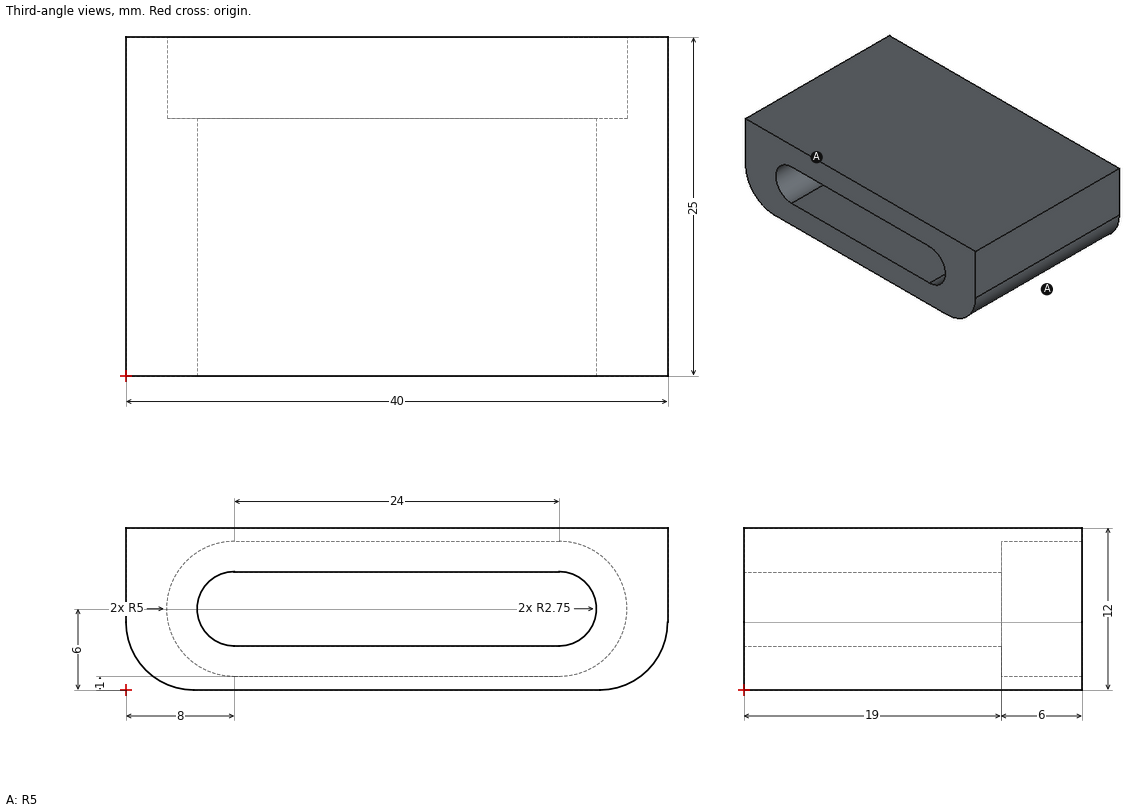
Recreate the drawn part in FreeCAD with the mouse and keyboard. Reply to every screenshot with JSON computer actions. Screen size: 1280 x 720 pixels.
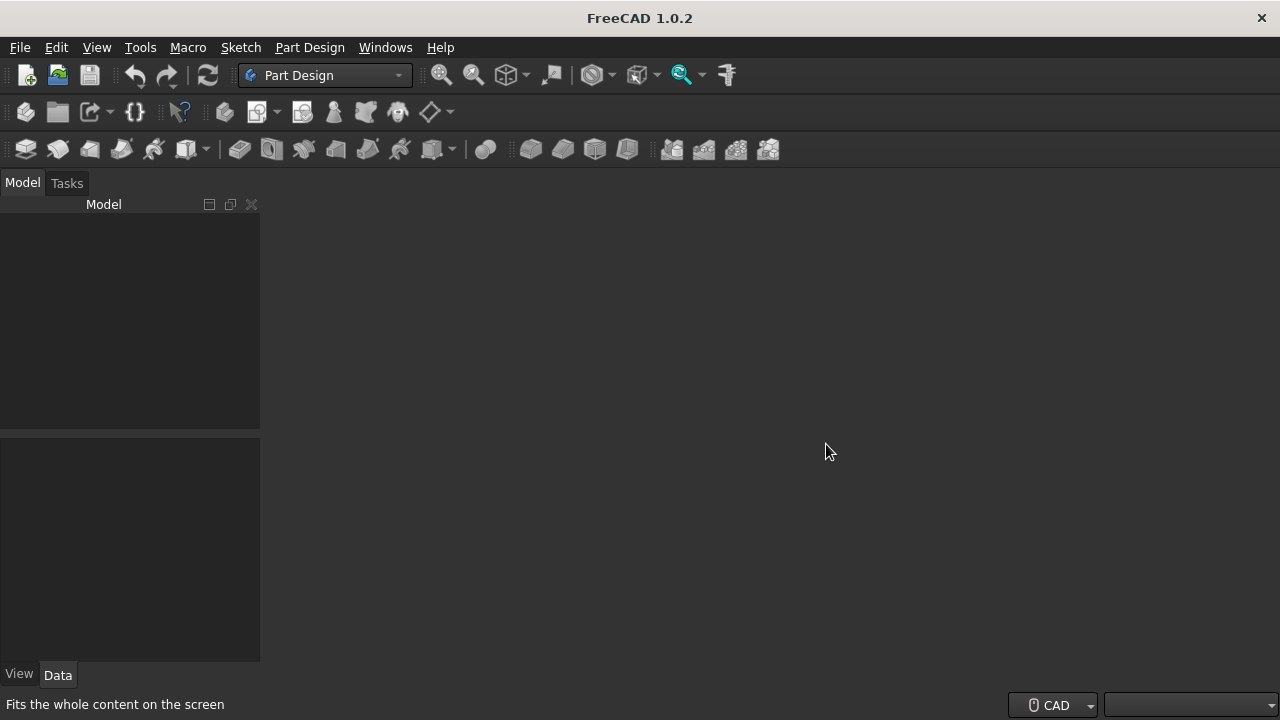
{"action": "key", "text": "ctrl+n"}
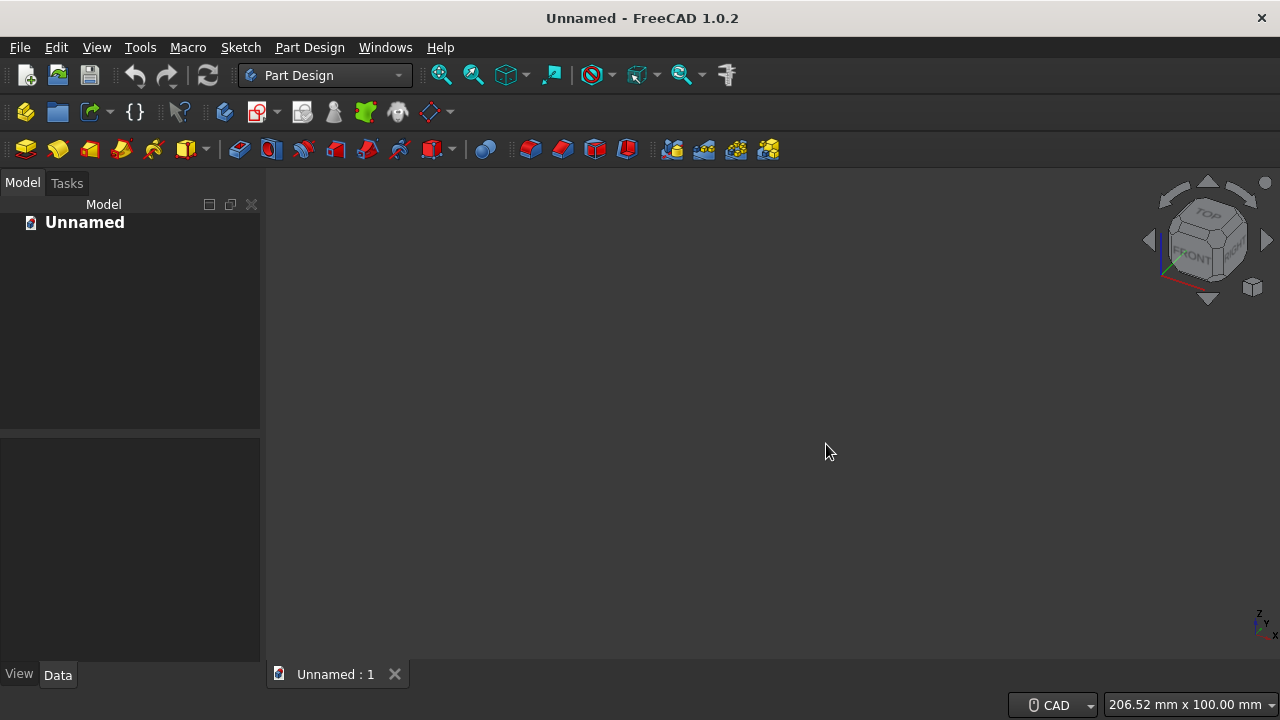
{"action": "left_click", "coordinate": [258, 112]}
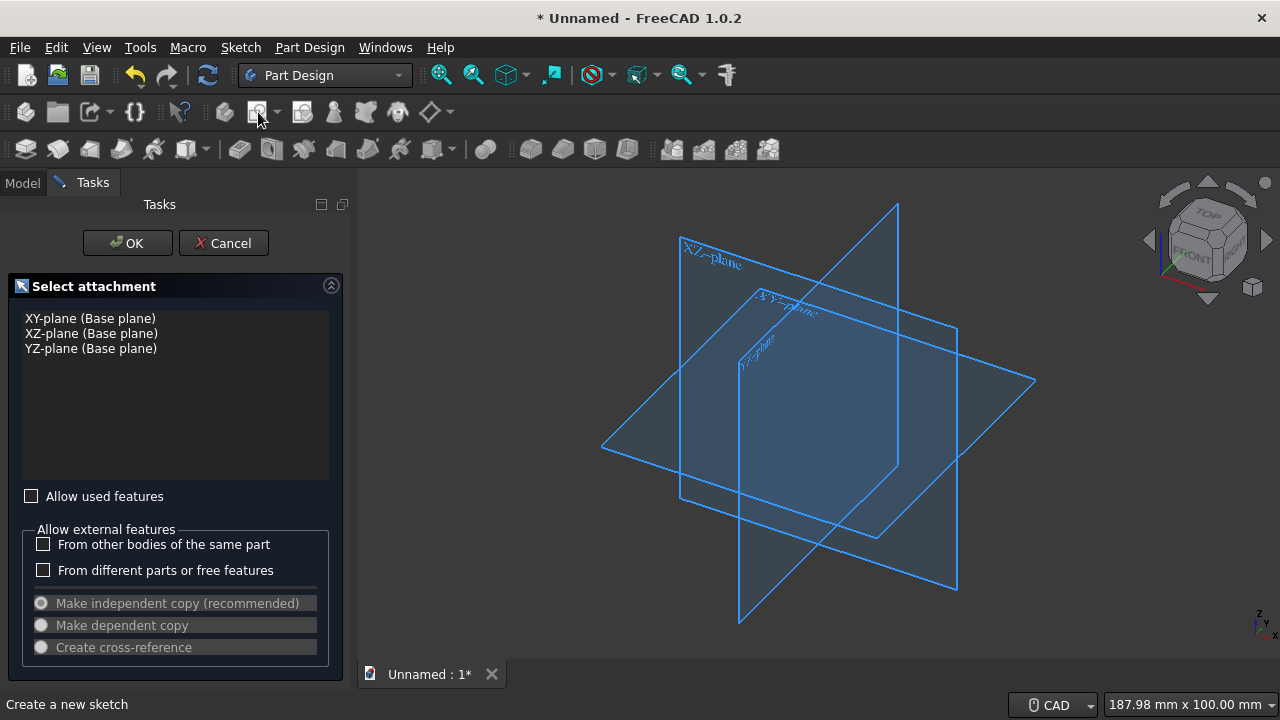
{"action": "left_click", "coordinate": [82, 318]}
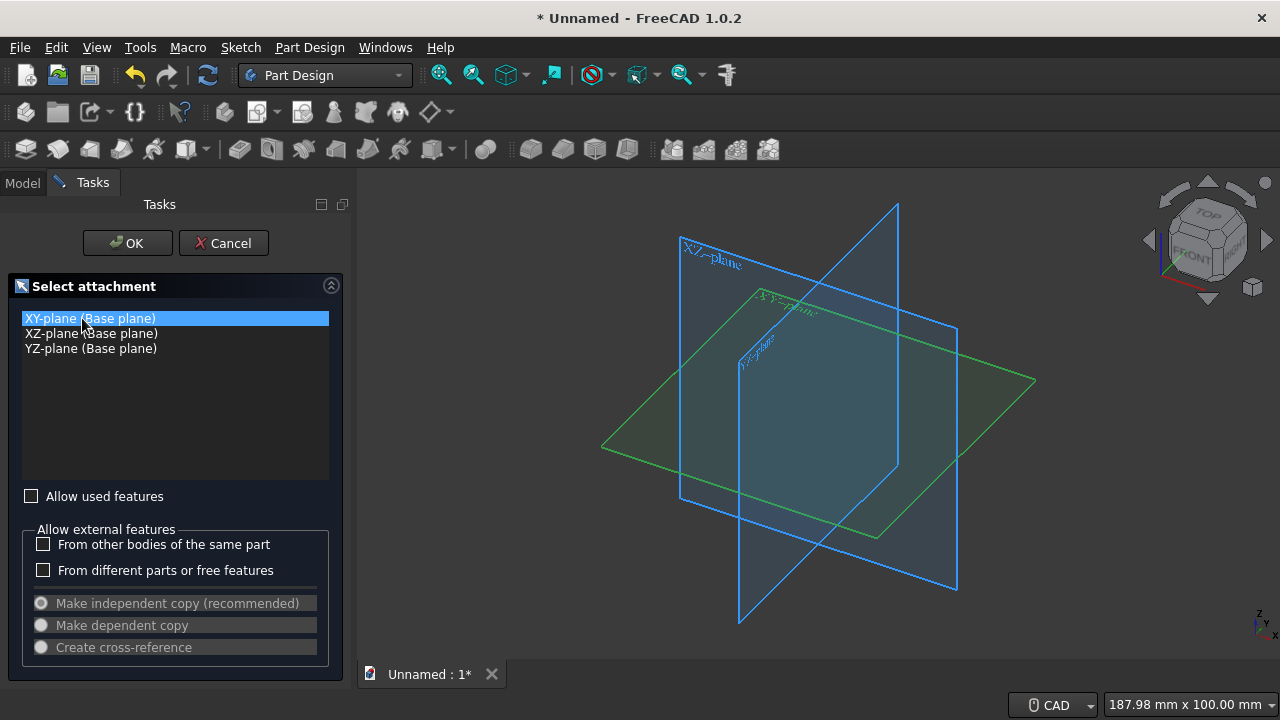
{"action": "left_click", "coordinate": [128, 243]}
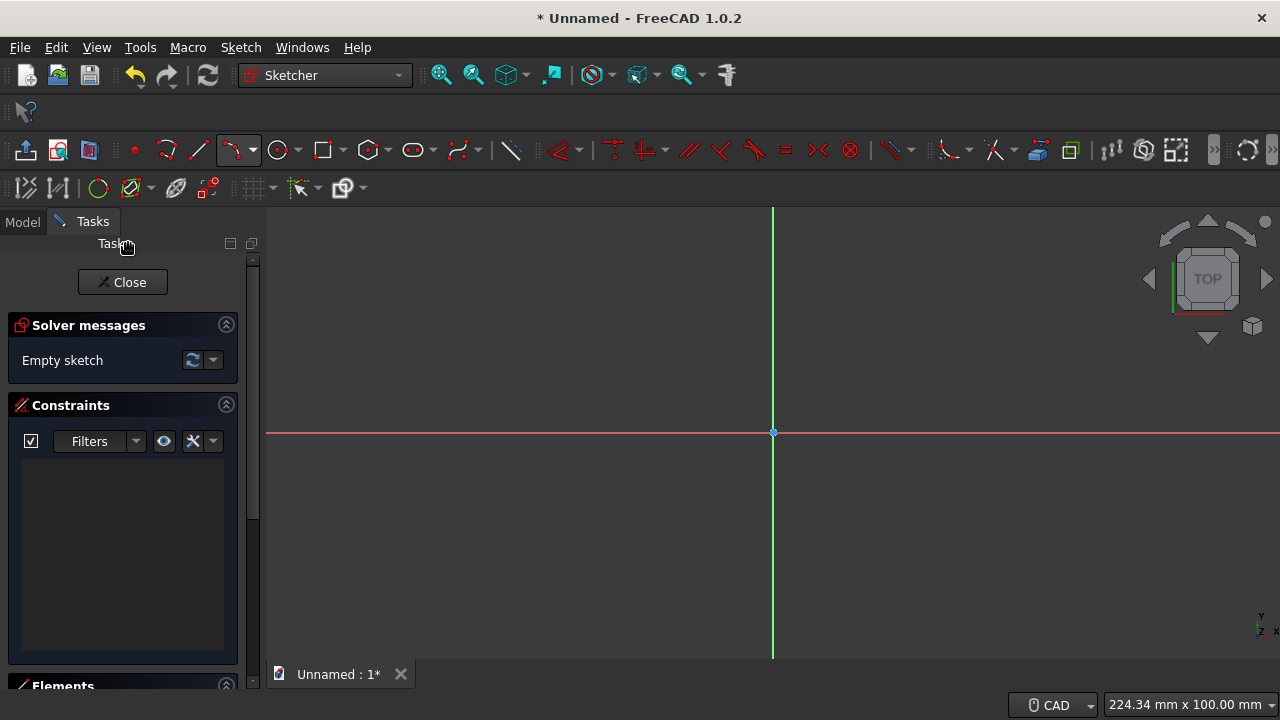
{"action": "scroll", "coordinate": [956, 344], "scroll_direction": "up", "scroll_amount": 5}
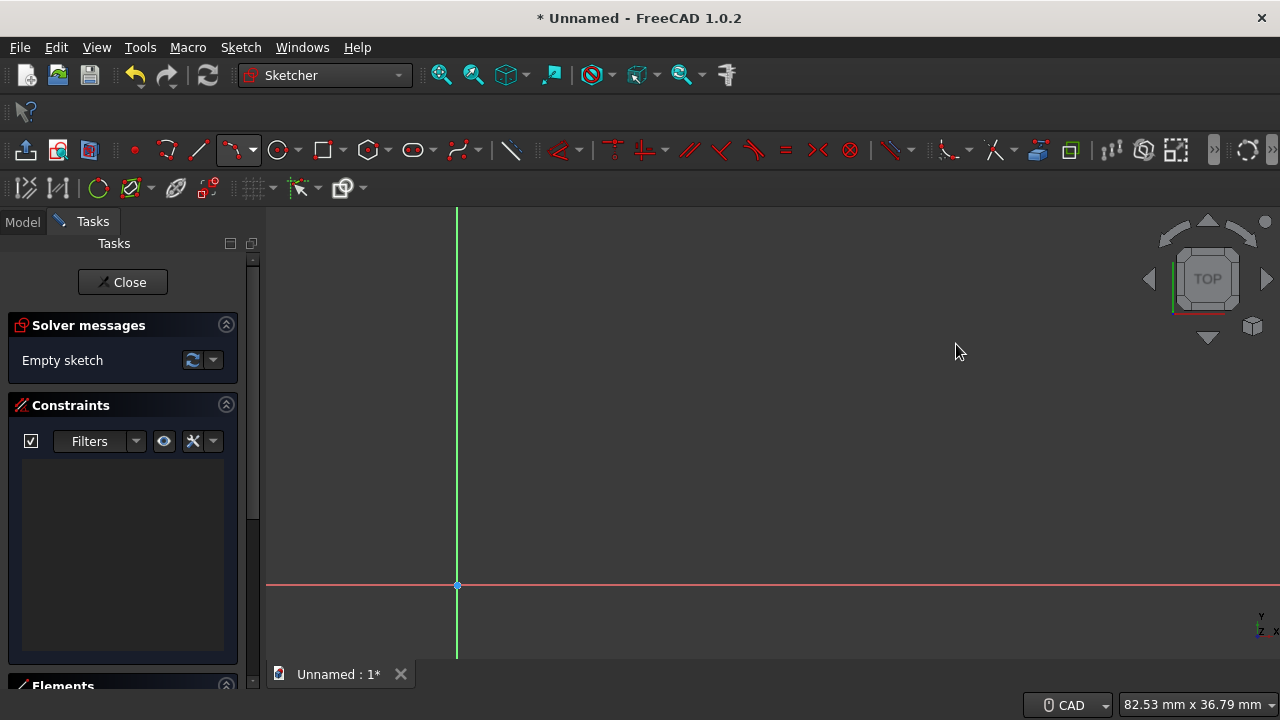
{"action": "key", "text": "g r"}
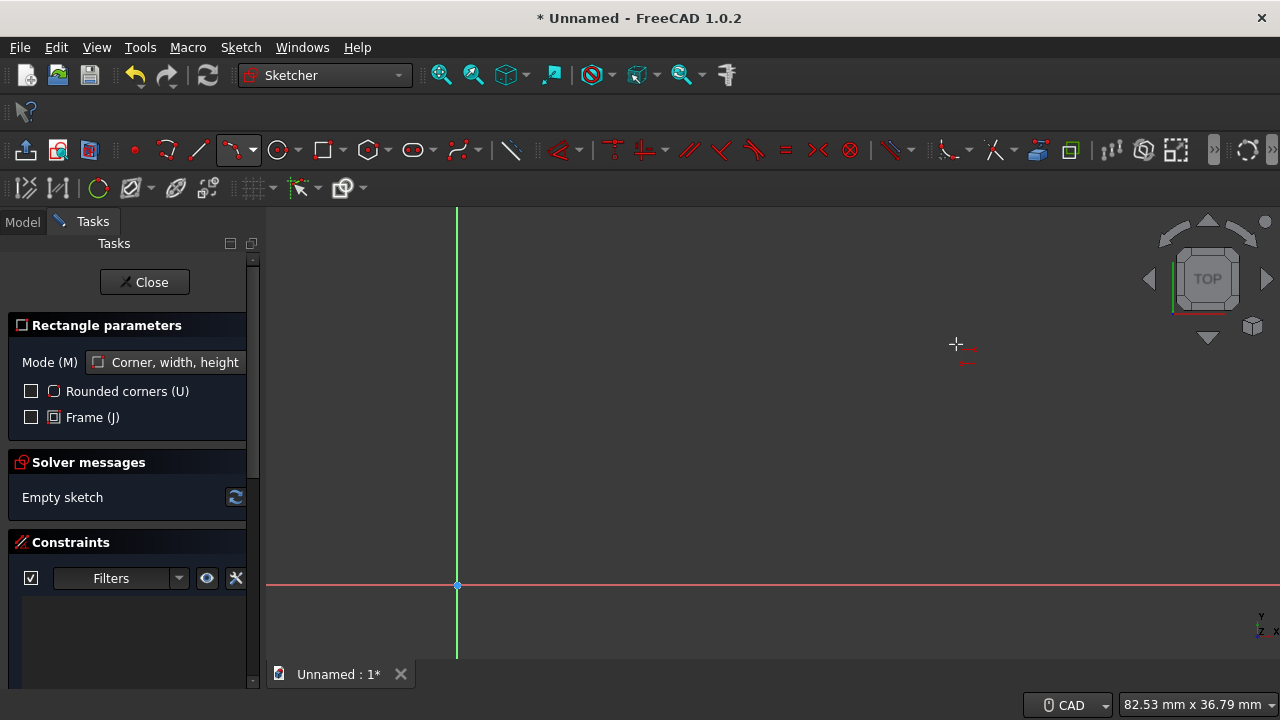
{"action": "left_click", "coordinate": [457, 585]}
{"action": "mouse_move", "coordinate": [949, 278]}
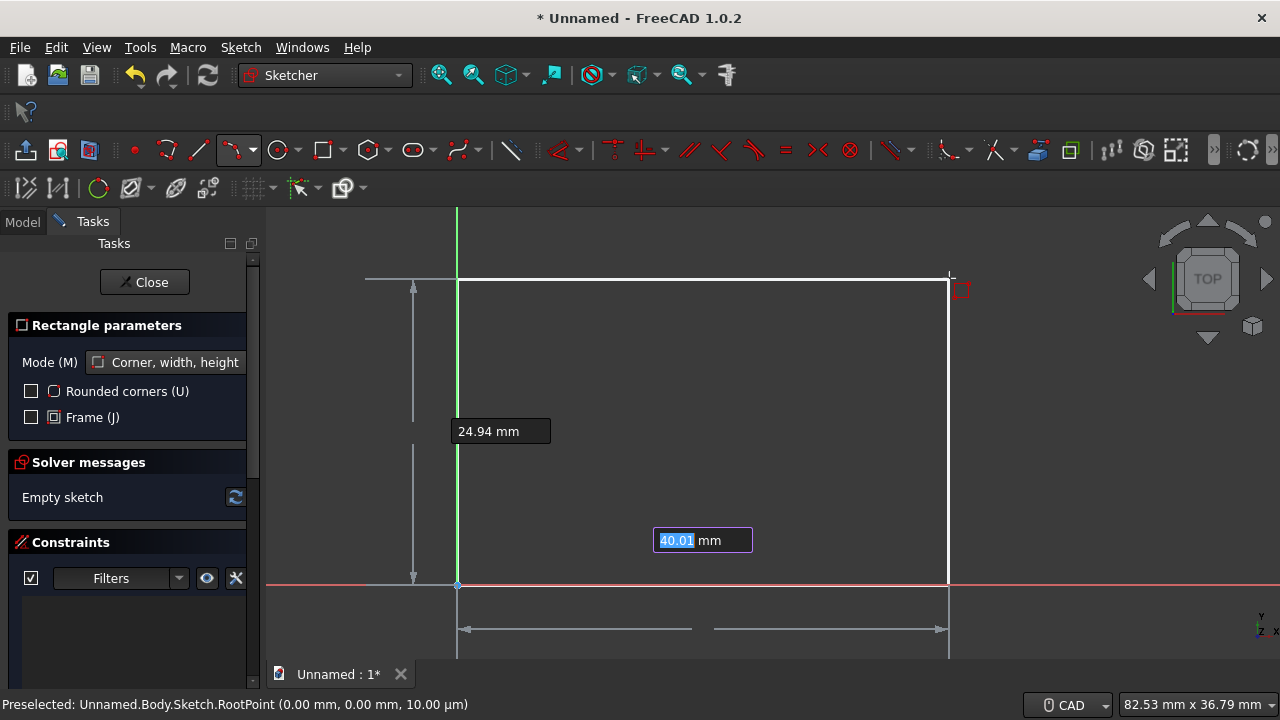
{"action": "type", "text": "40"}
{"action": "key", "text": "Tab"}
{"action": "type", "text": "25"}
{"action": "key", "text": "Return"}
{"action": "key", "text": "Escape"}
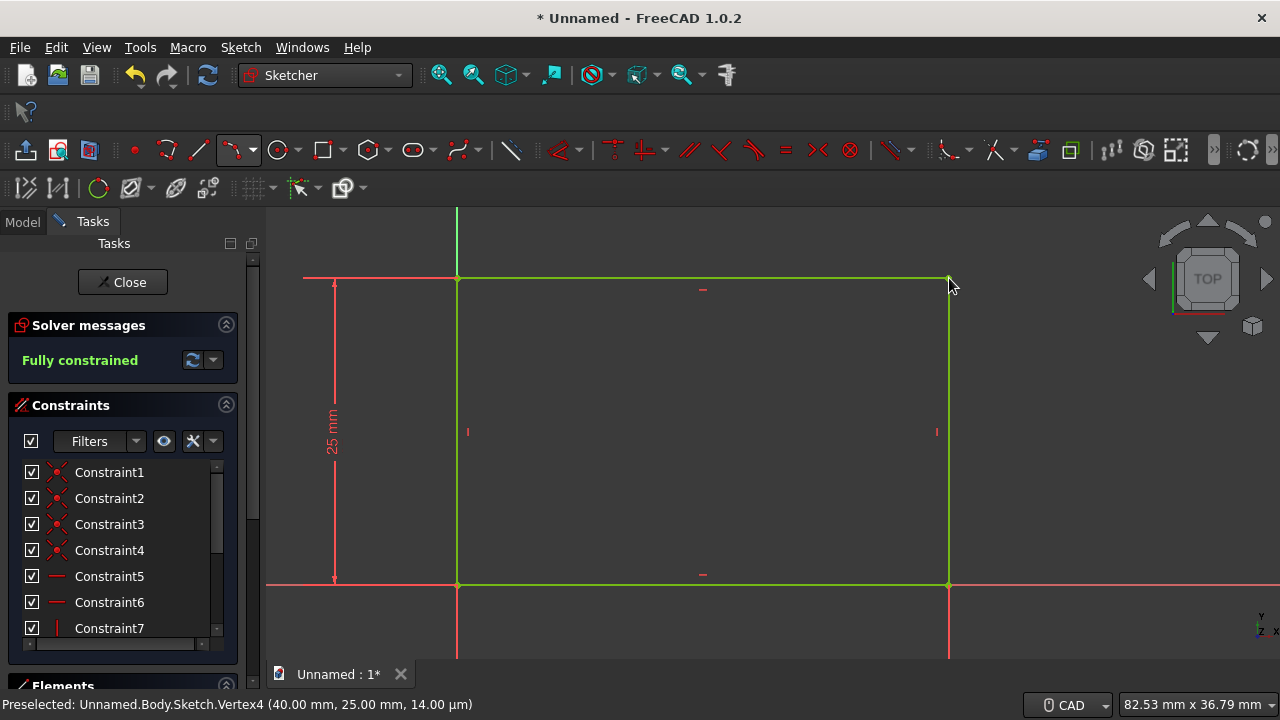
{"action": "left_click", "coordinate": [123, 282]}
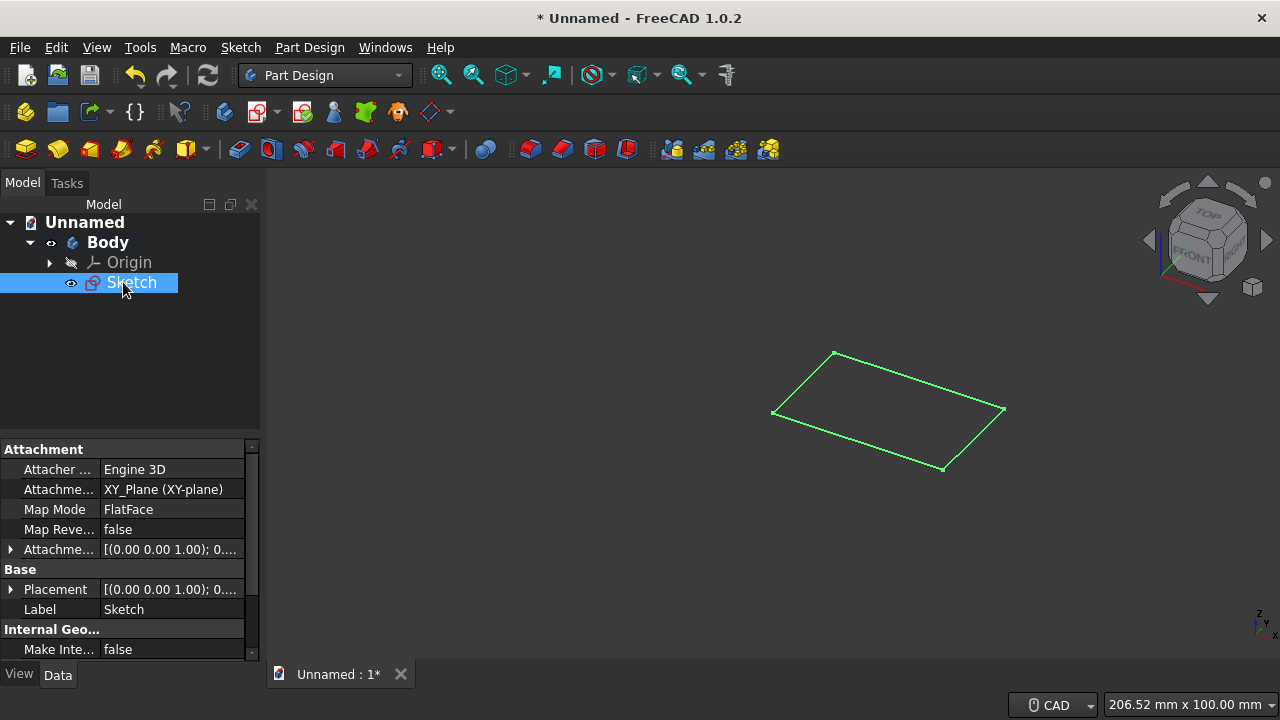
{"action": "left_click", "coordinate": [26, 150]}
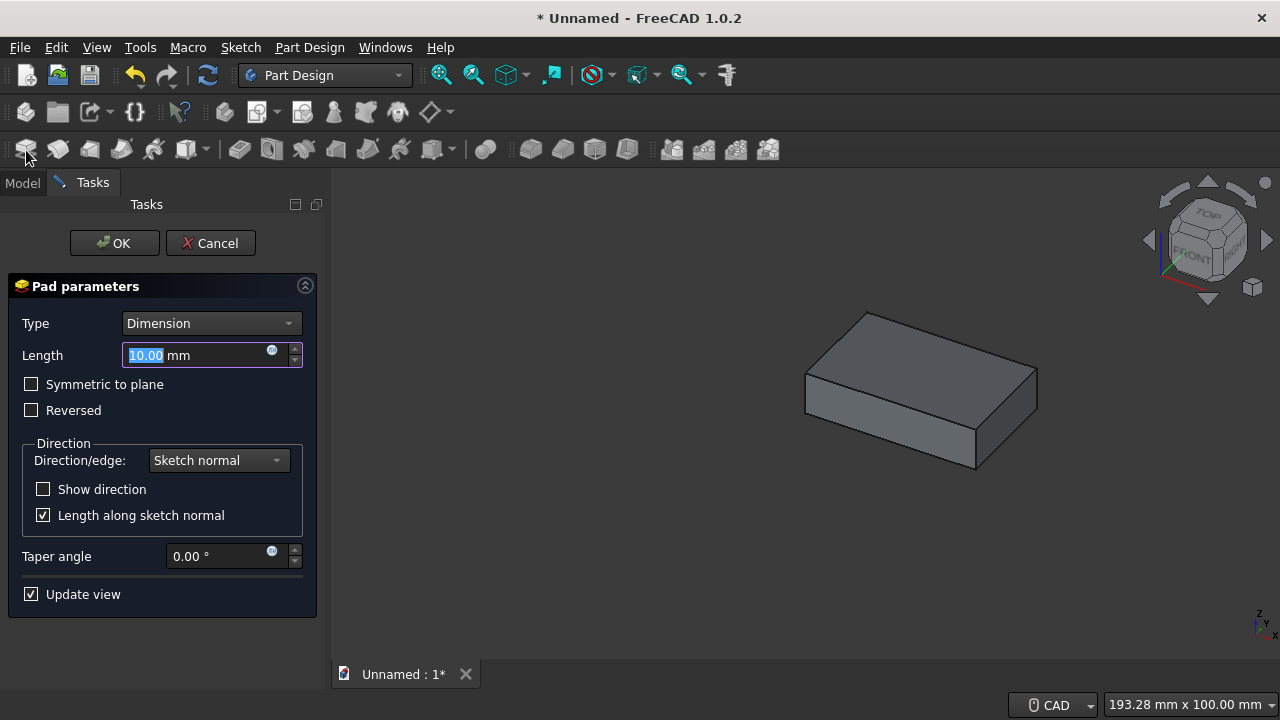
{"action": "type", "text": "12"}
{"action": "key", "text": "Tab"}